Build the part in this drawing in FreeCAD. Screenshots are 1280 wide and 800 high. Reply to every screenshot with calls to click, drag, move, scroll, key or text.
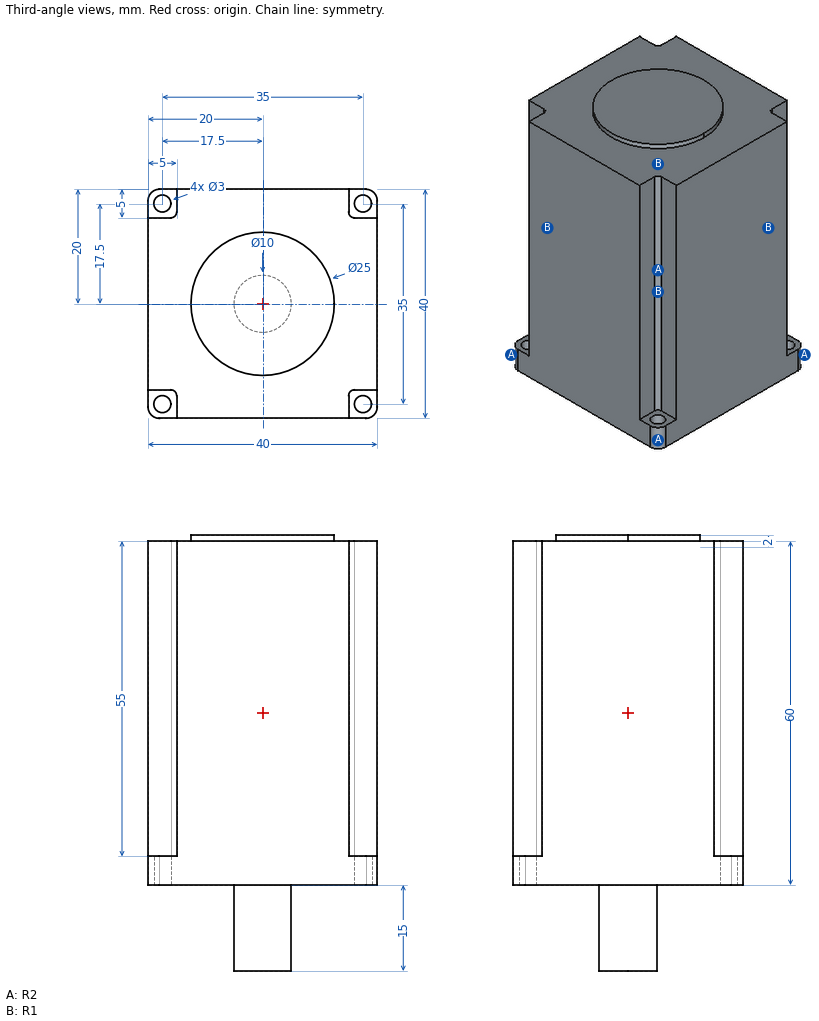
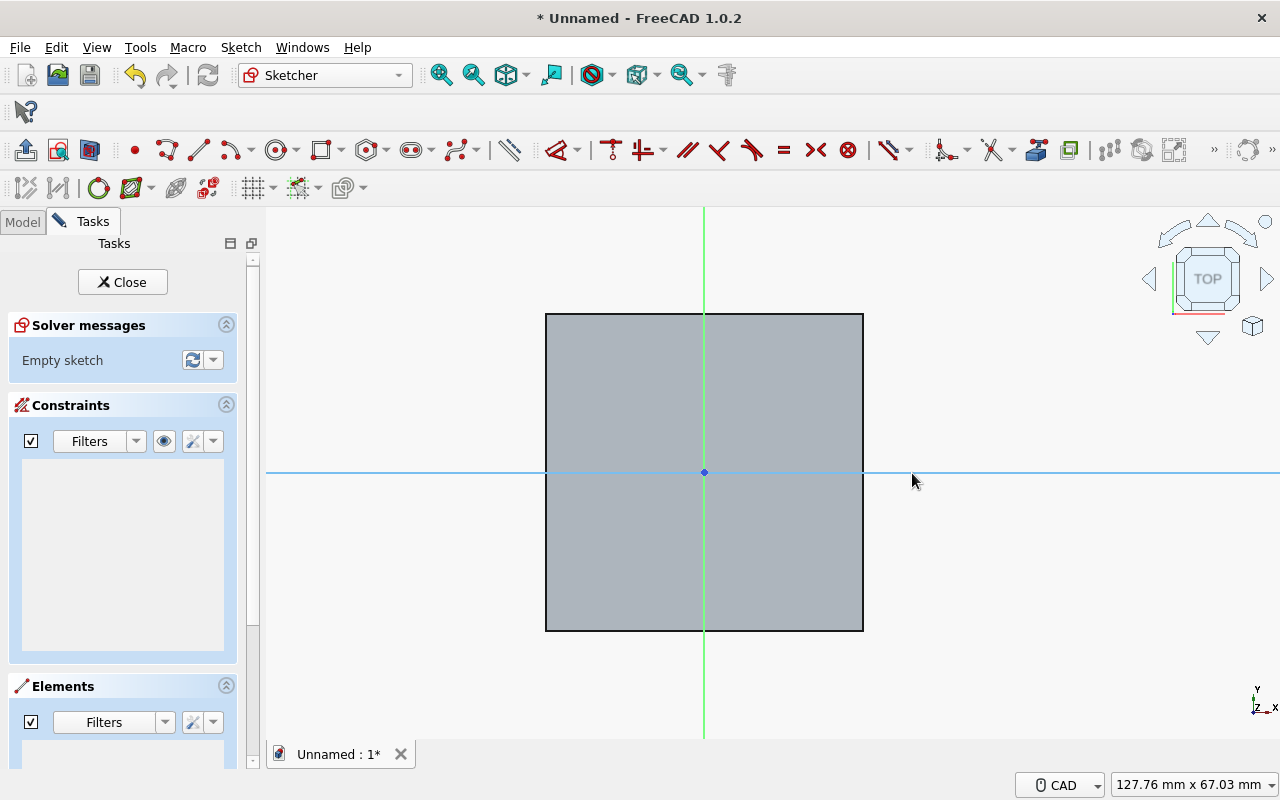
click(322, 150)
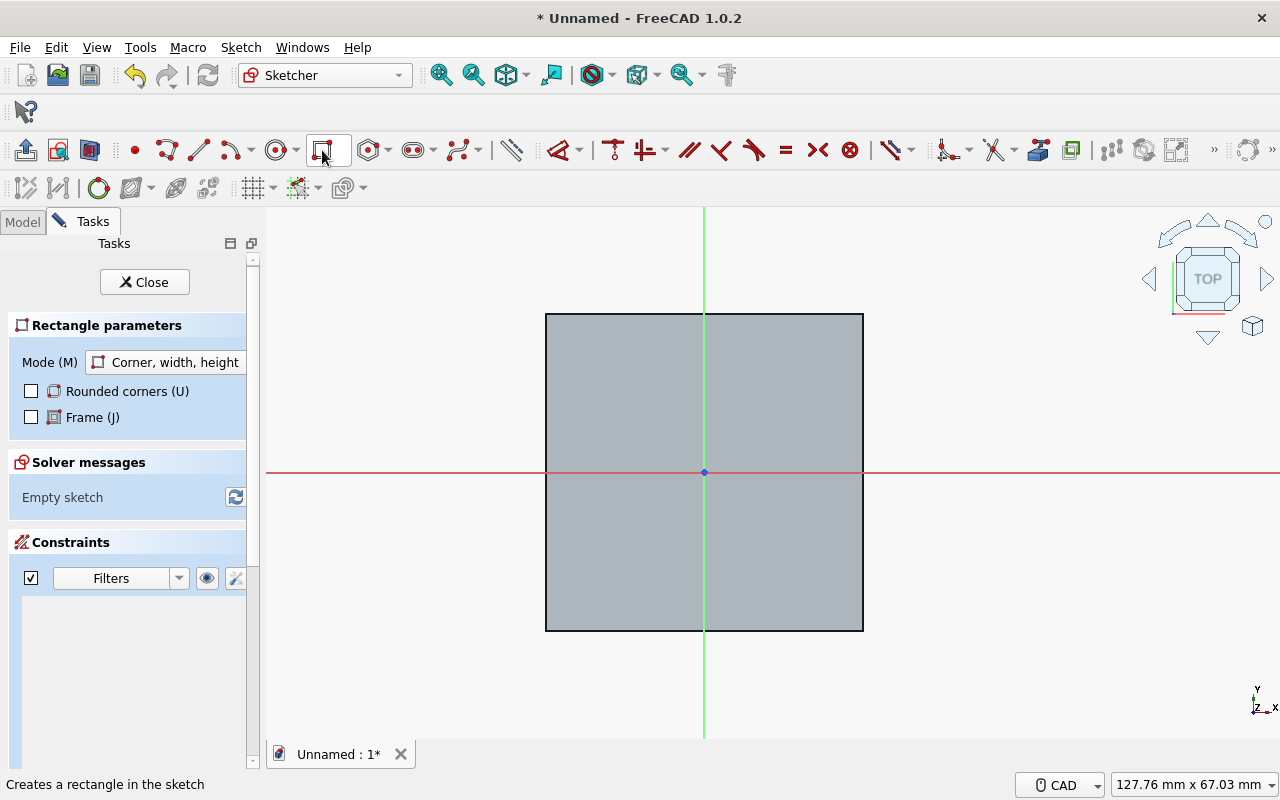
click(546, 314)
click(585, 354)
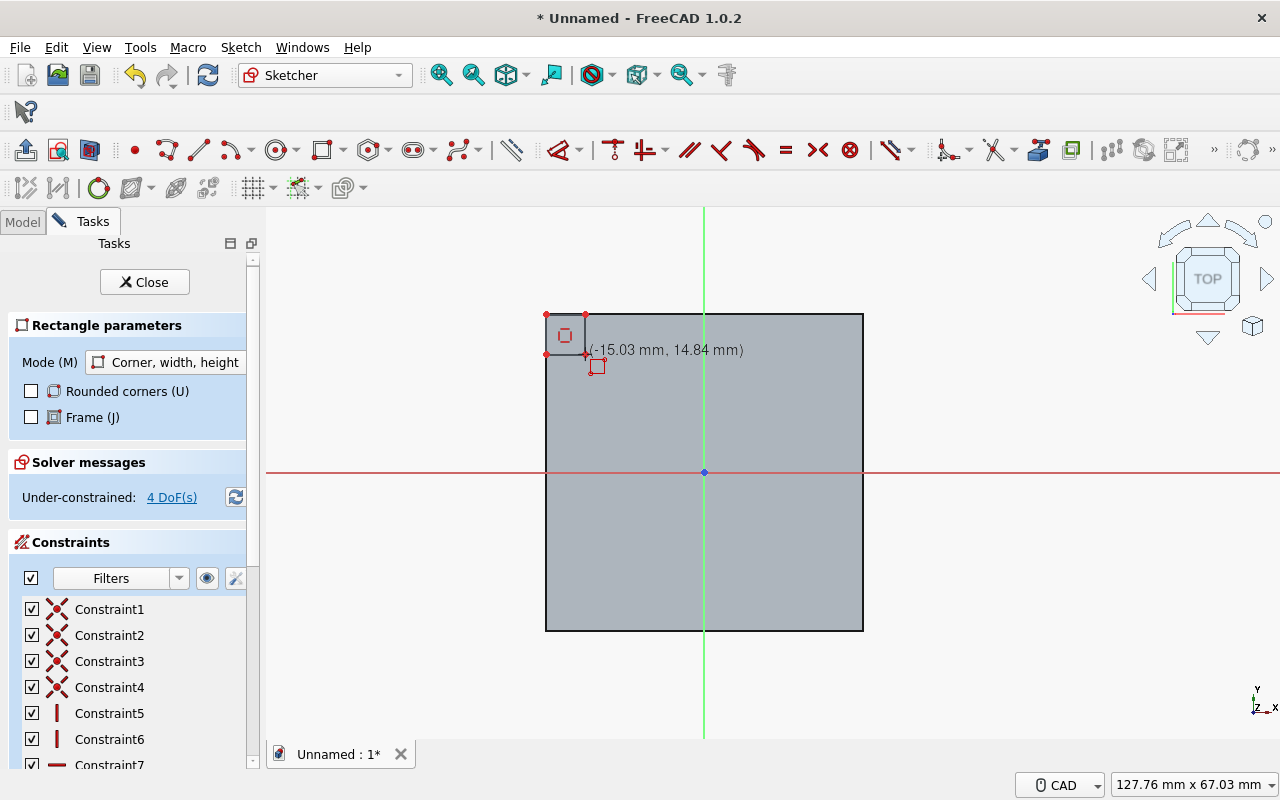
click(823, 314)
click(863, 354)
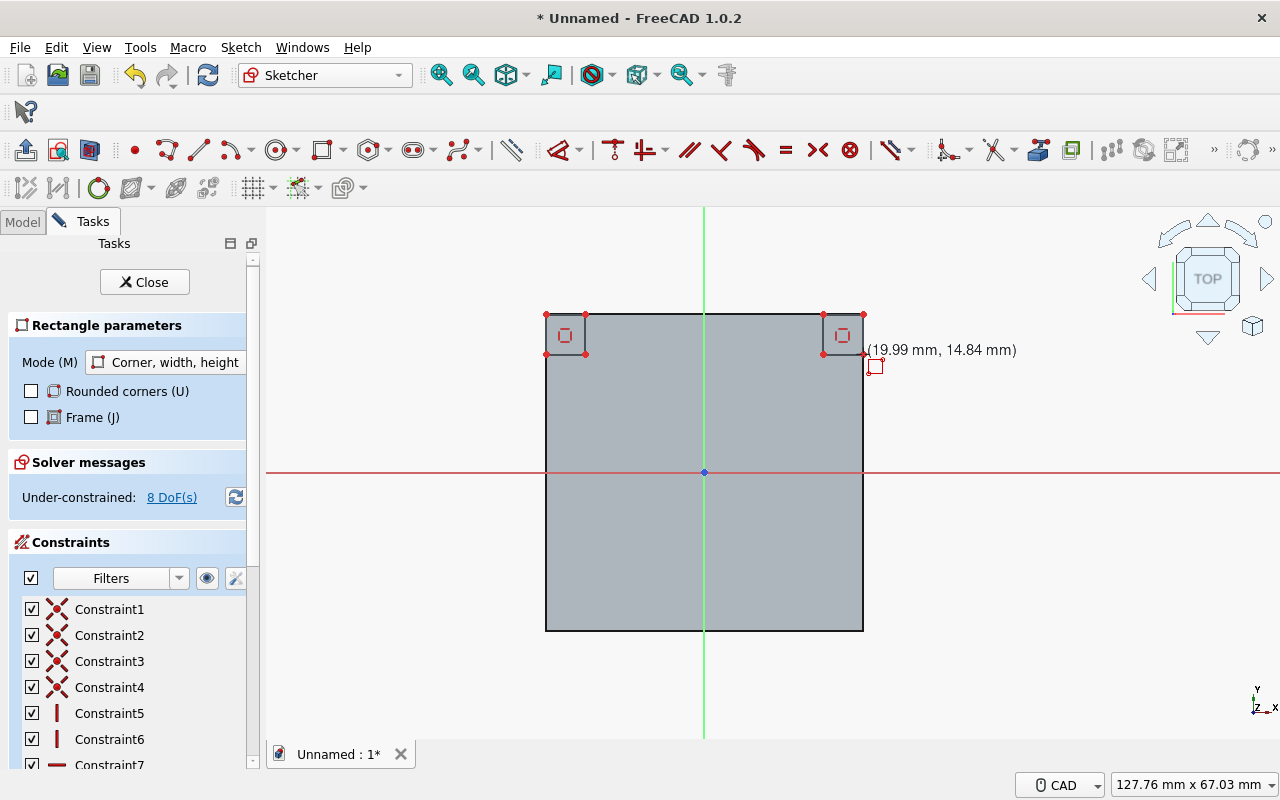
click(823, 592)
click(863, 631)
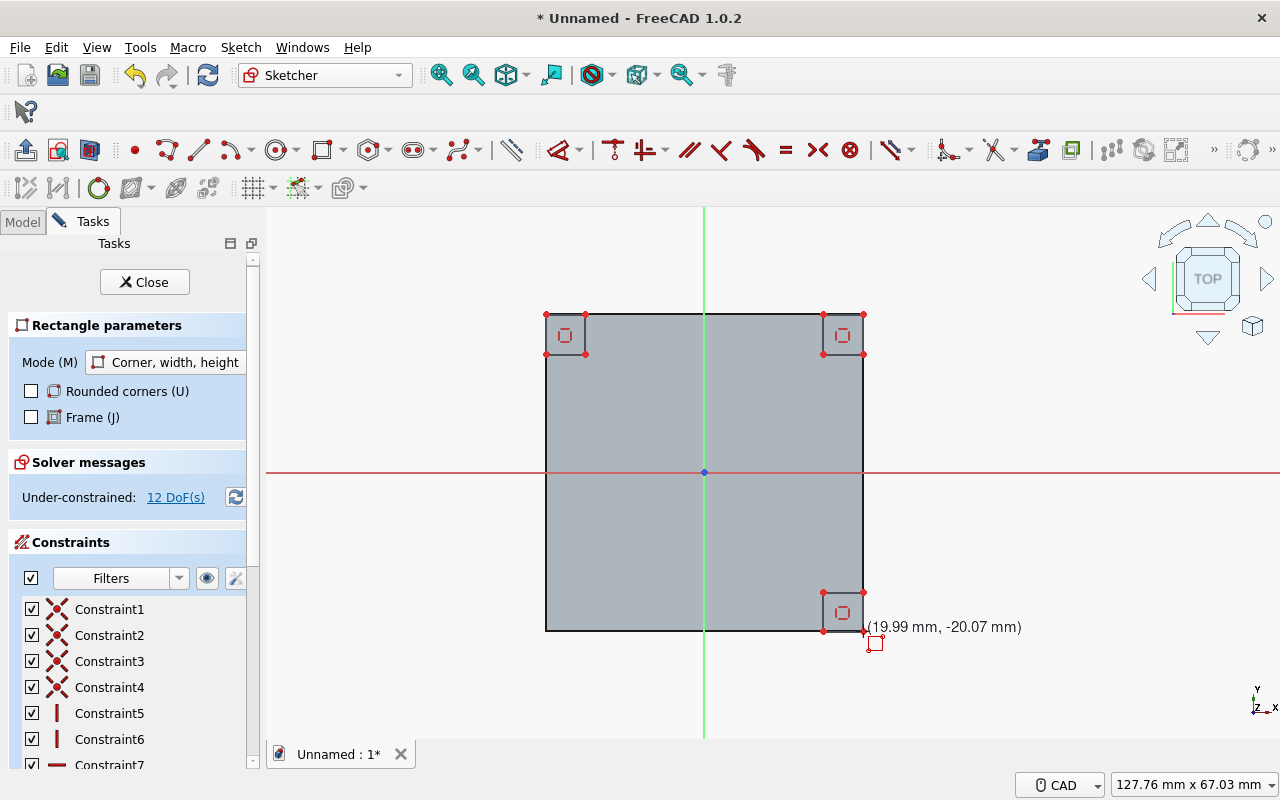
click(546, 592)
click(585, 631)
key(Escape)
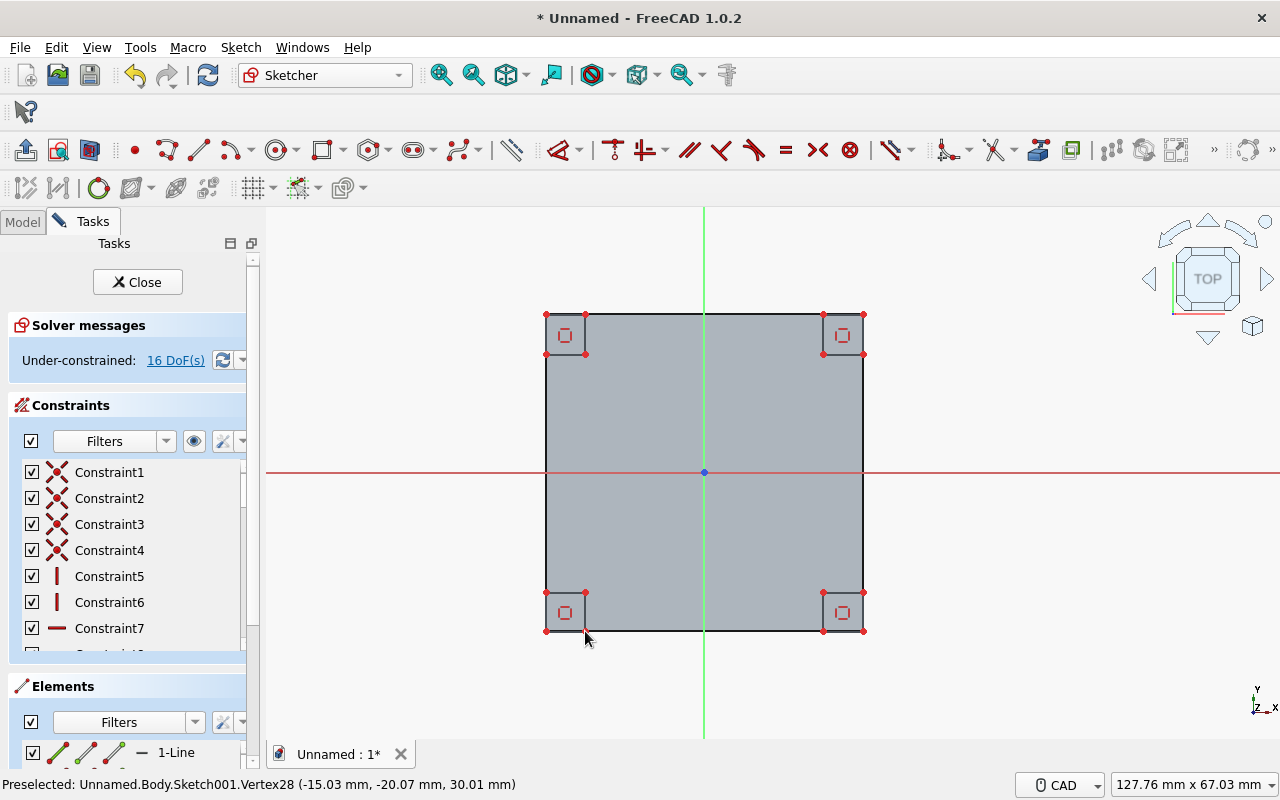
click(585, 315)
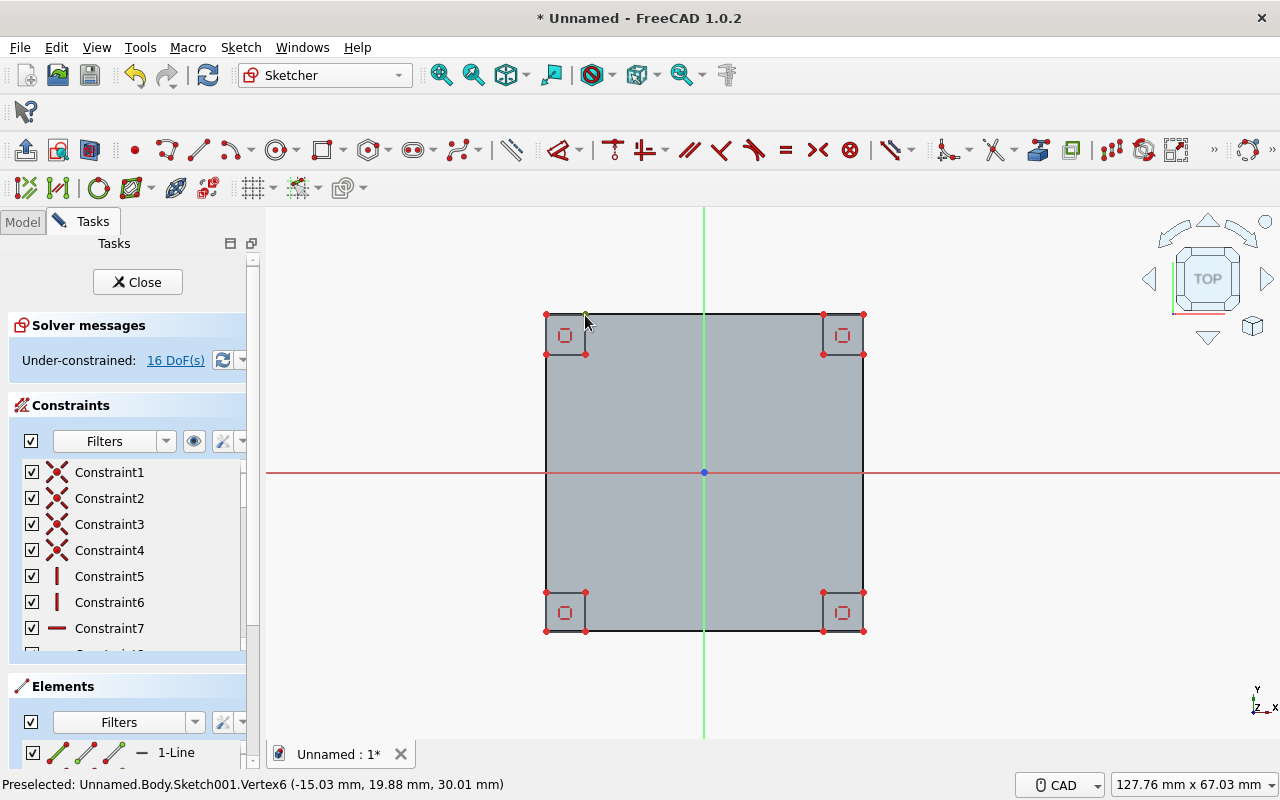
click(823, 315)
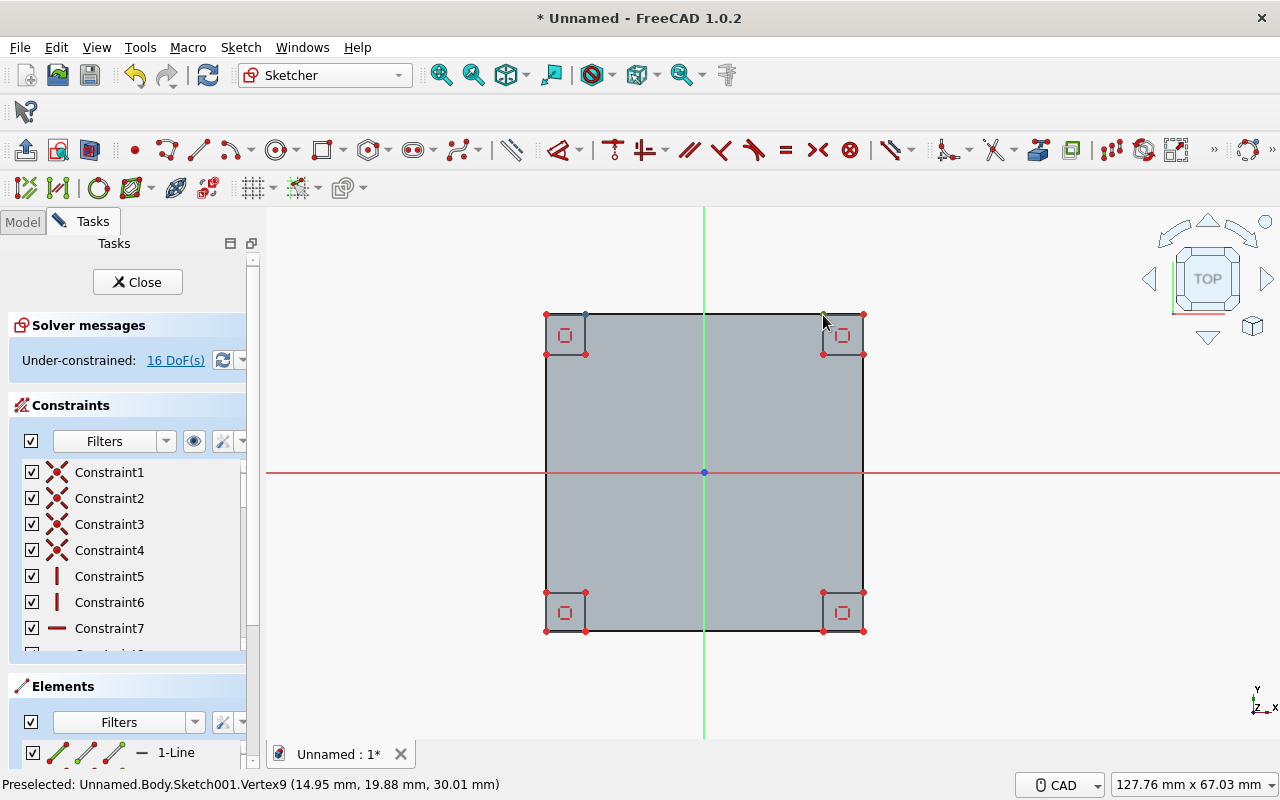
click(704, 677)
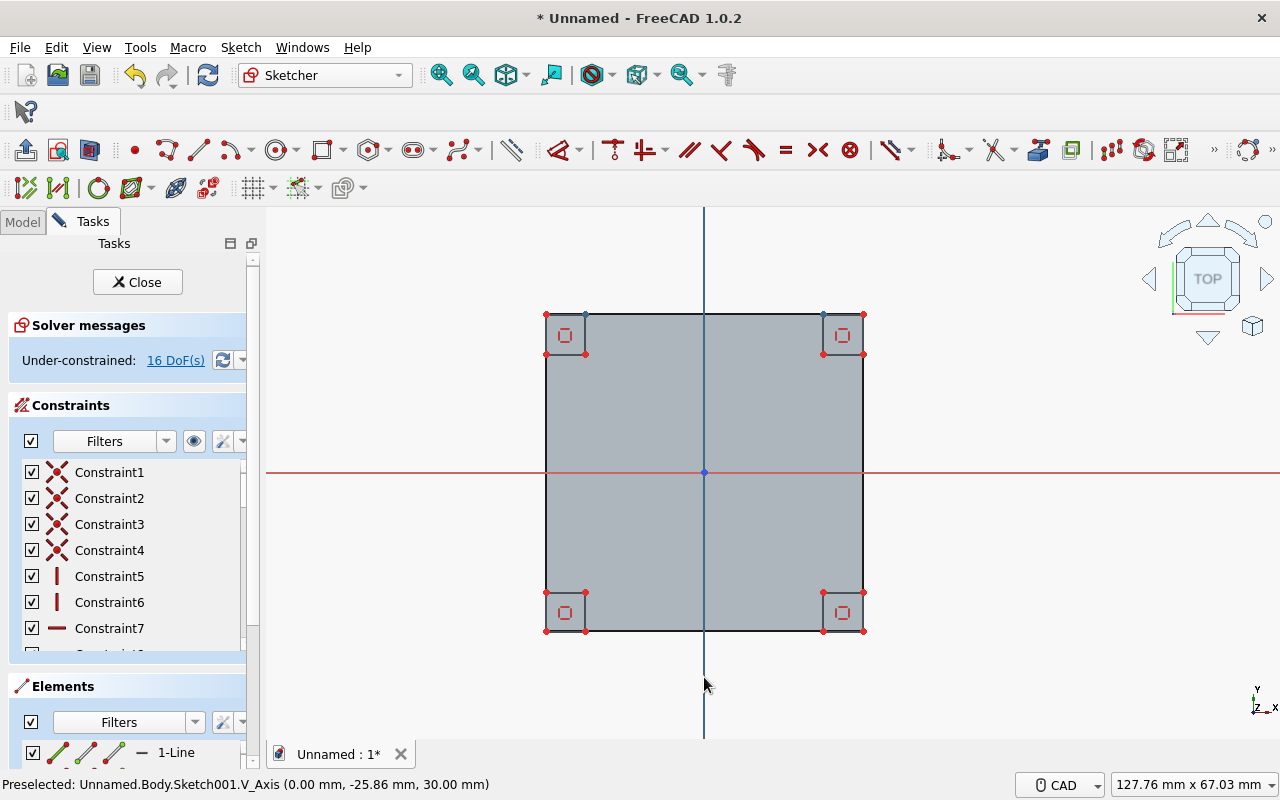
click(818, 150)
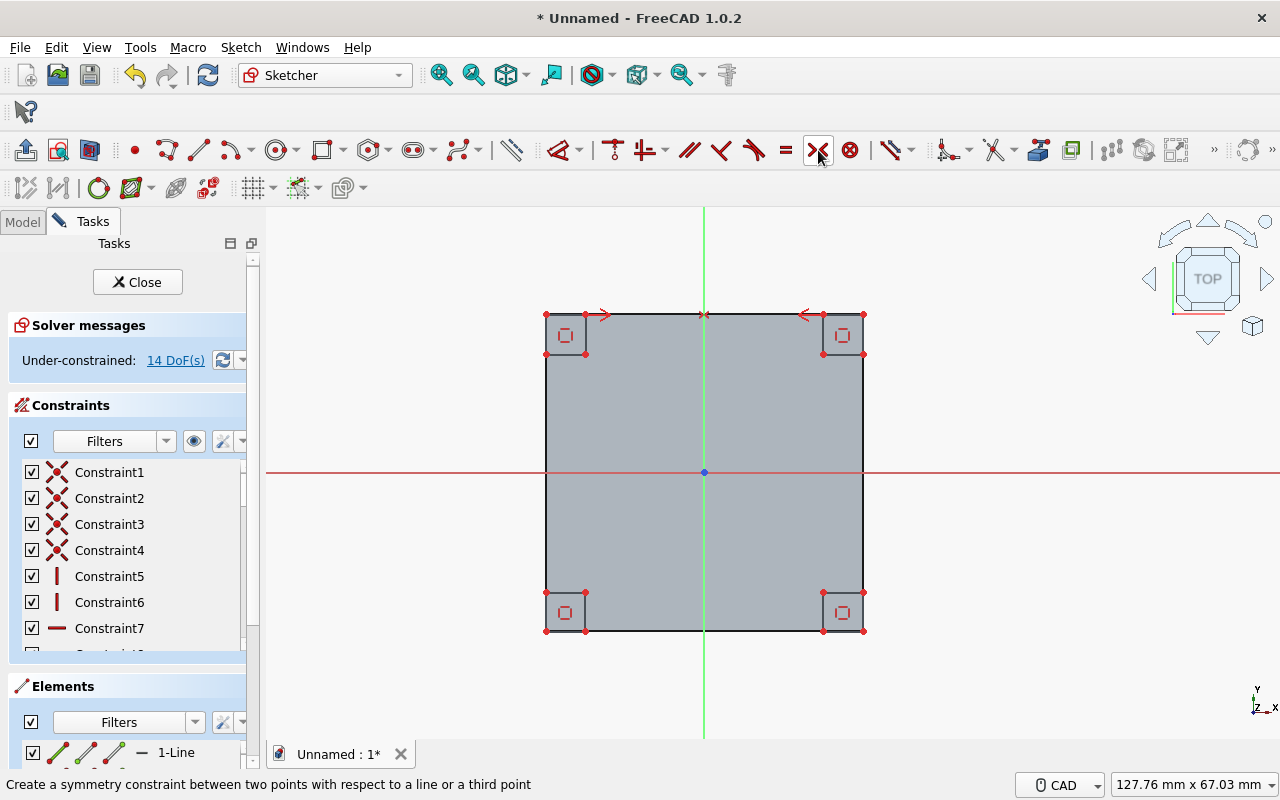
click(546, 355)